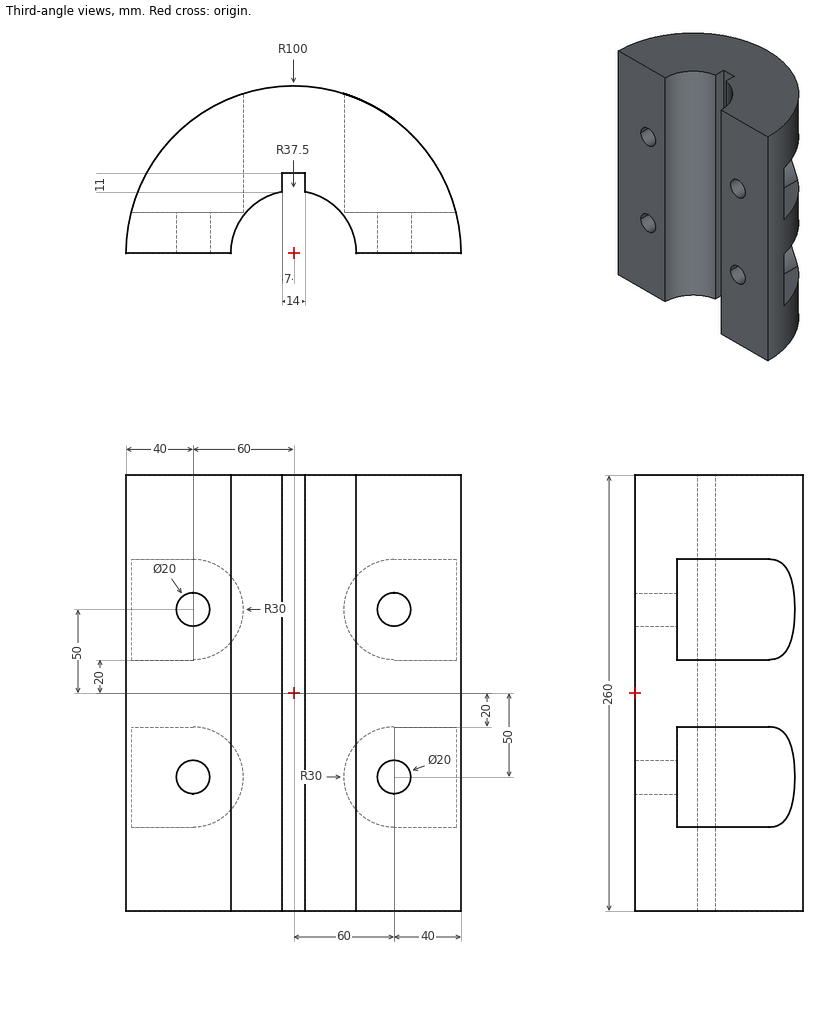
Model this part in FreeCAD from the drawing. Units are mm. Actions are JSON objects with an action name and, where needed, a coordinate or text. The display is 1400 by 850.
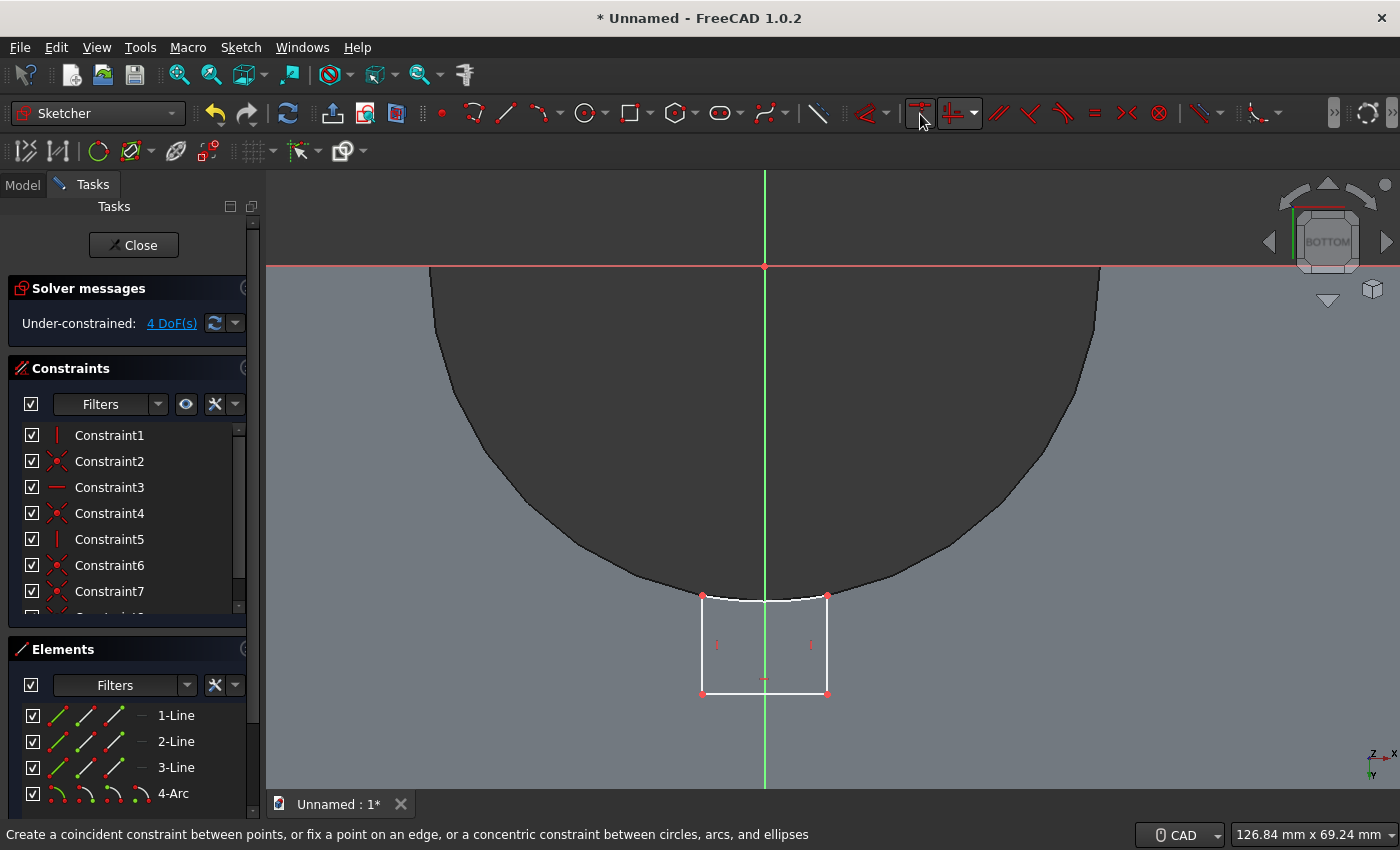
{"action": "left_click", "coordinate": [866, 114]}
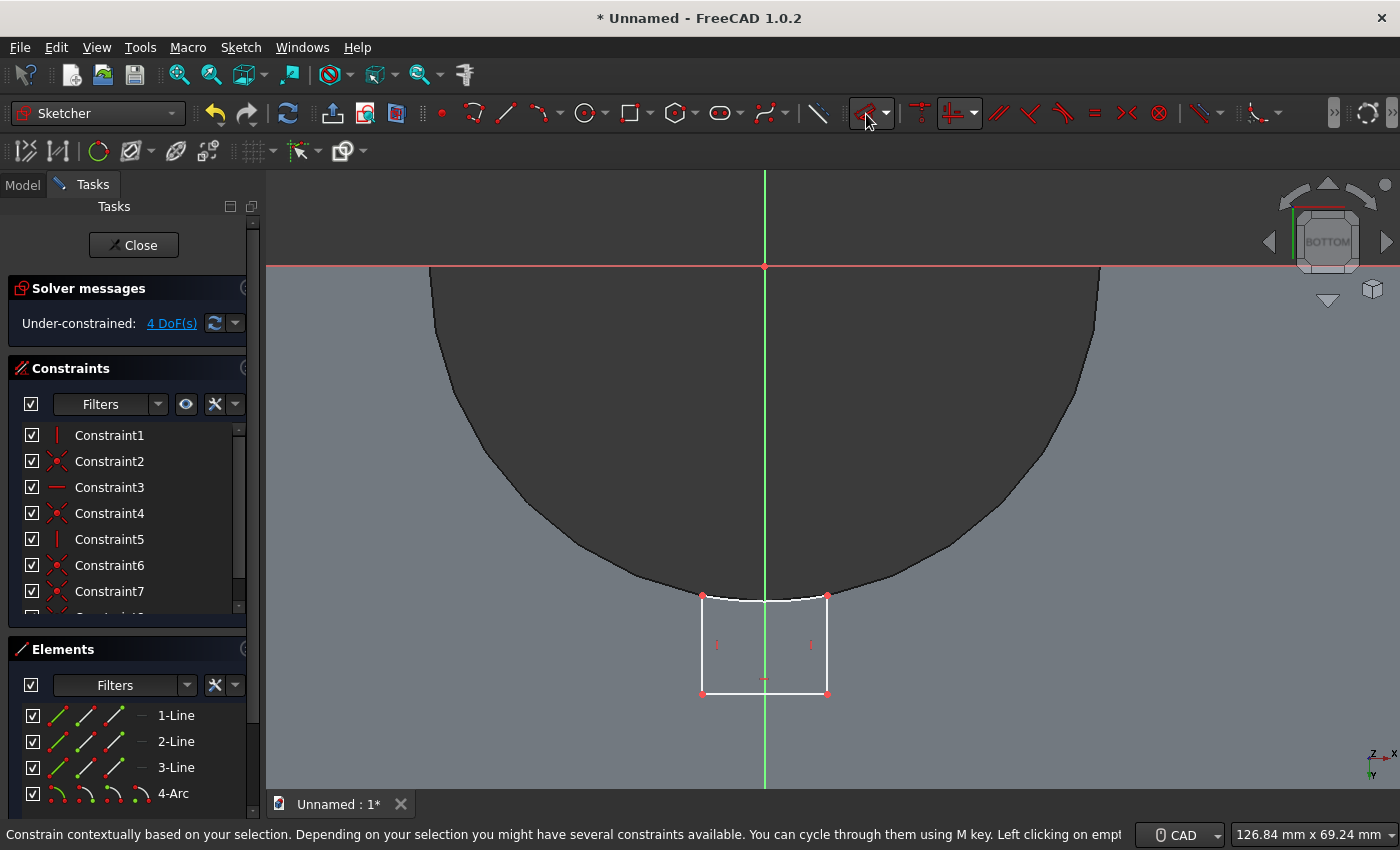
{"action": "left_click", "coordinate": [739, 601]}
{"action": "left_click", "coordinate": [737, 633]}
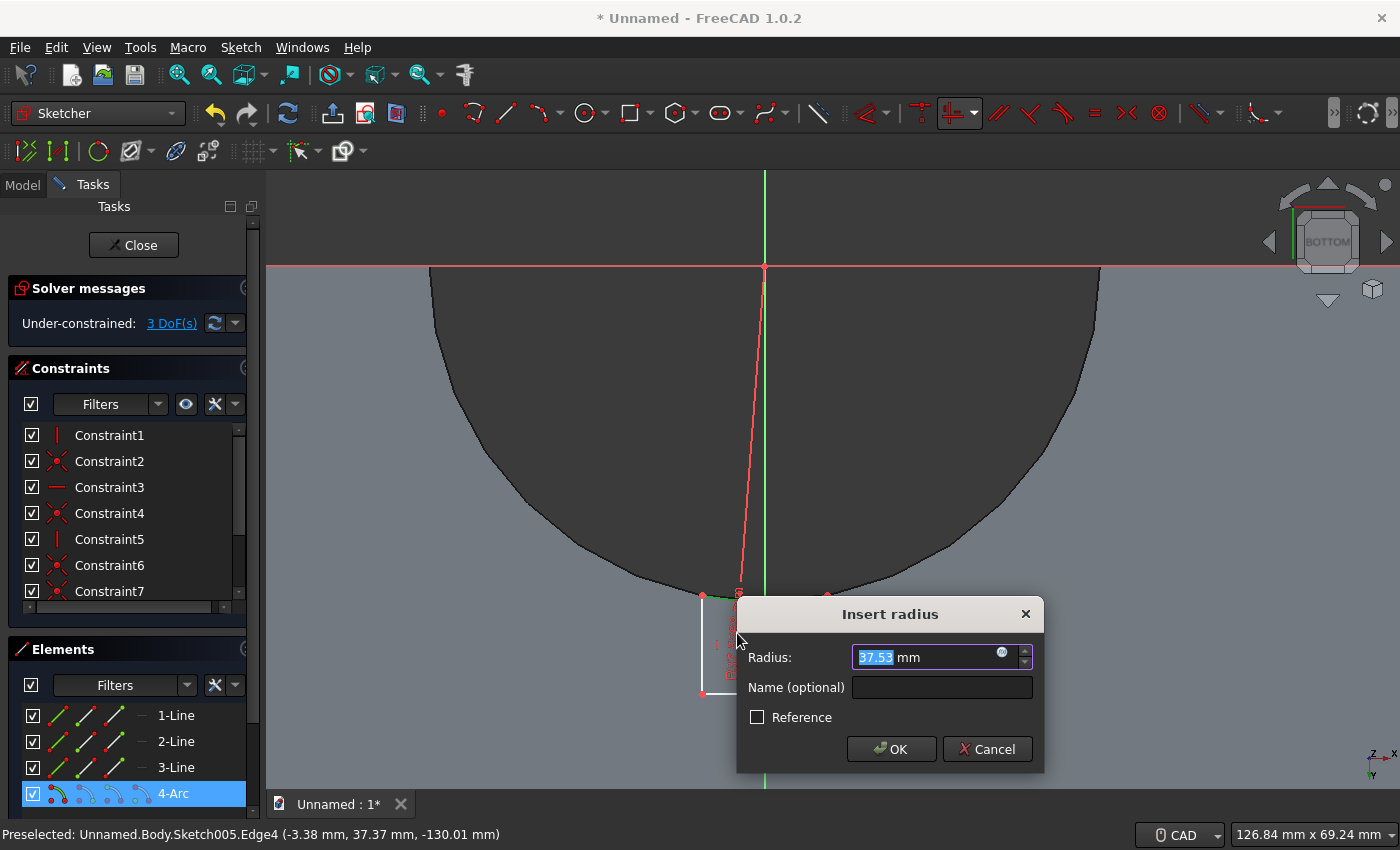
{"action": "type", "text": "37.5"}
{"action": "key", "text": "Return"}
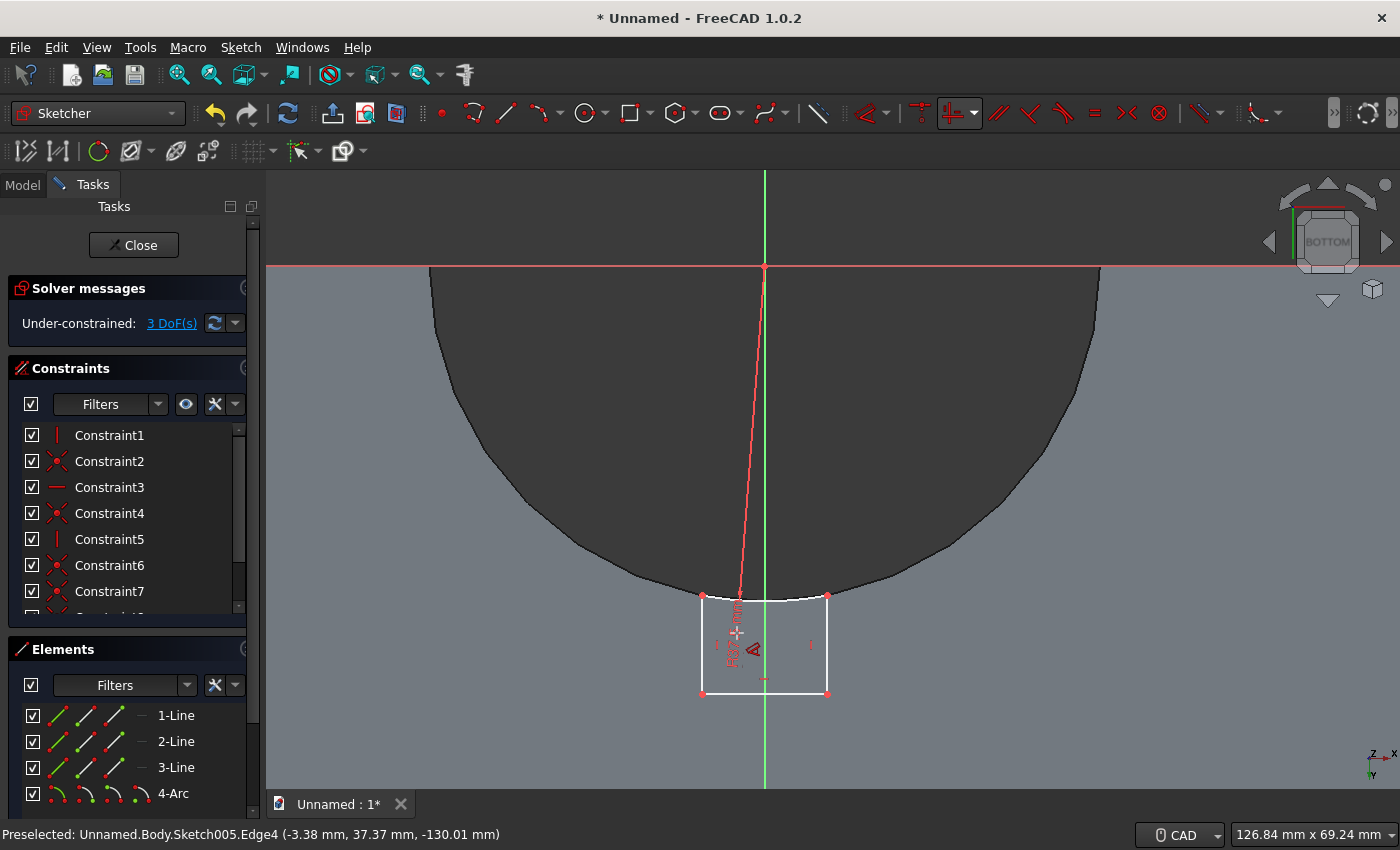
{"action": "left_click", "coordinate": [702, 625]}
{"action": "left_click", "coordinate": [668, 667]}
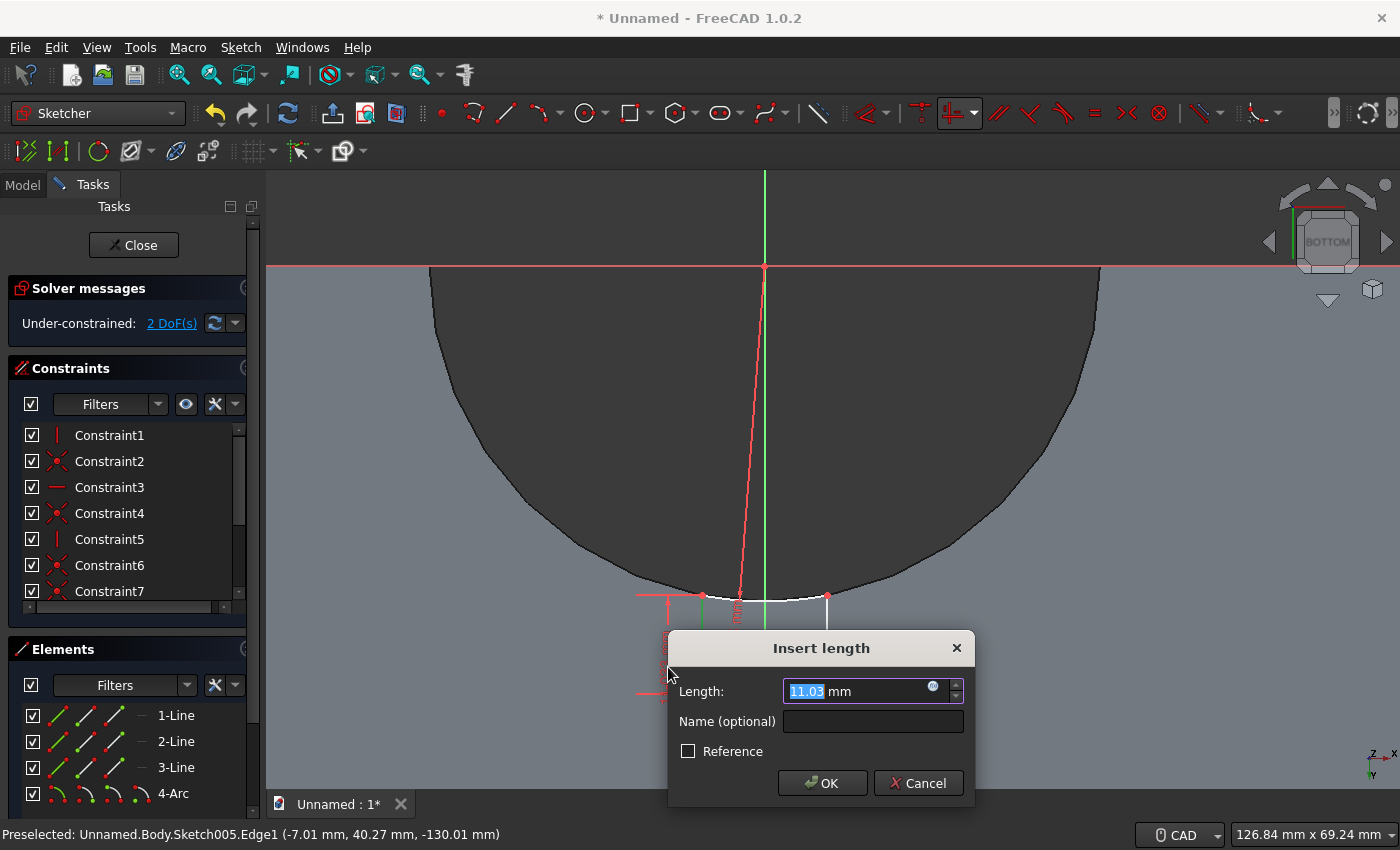
{"action": "type", "text": "11"}
{"action": "key", "text": "Return"}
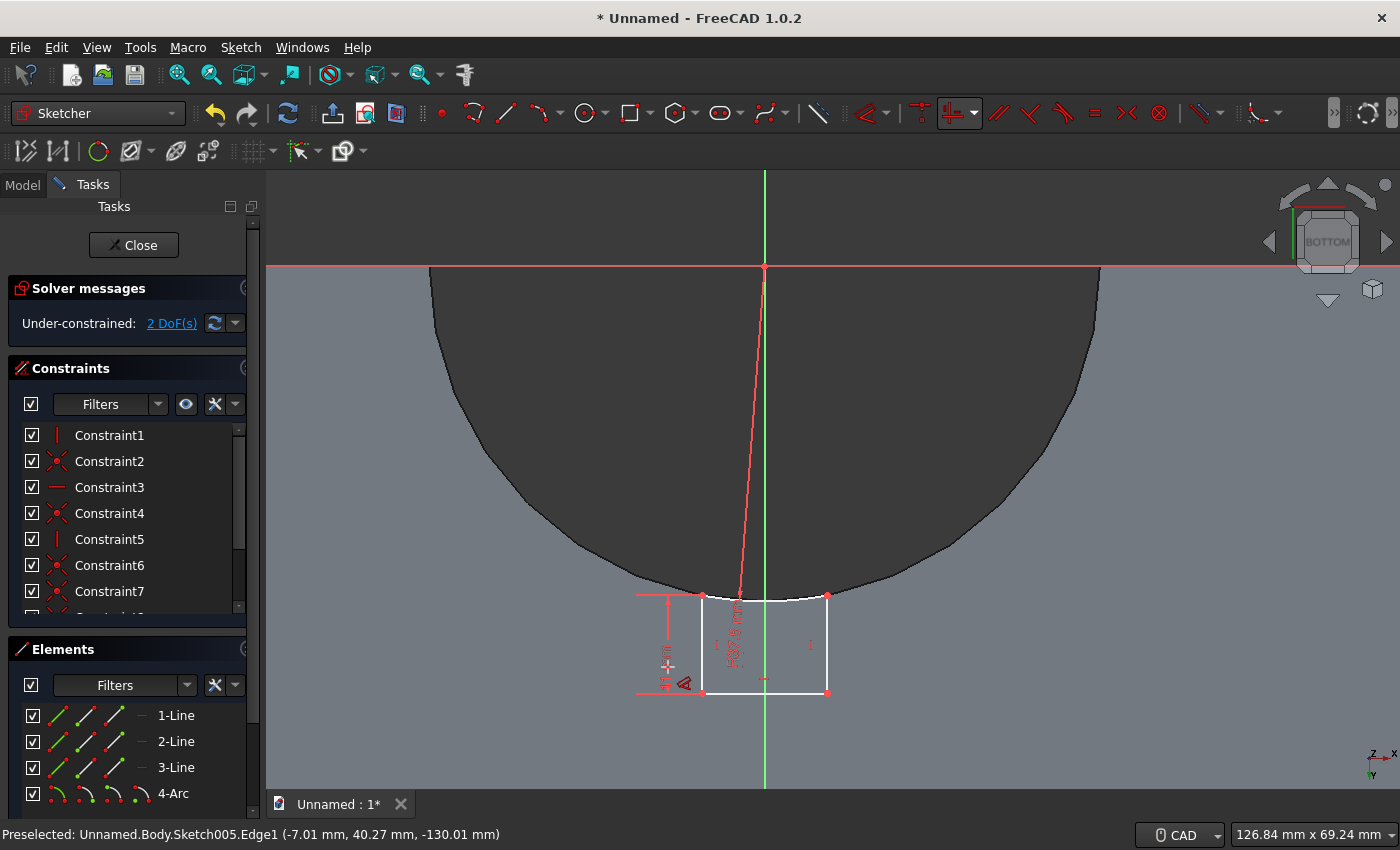
{"action": "left_click", "coordinate": [740, 694]}
{"action": "left_click", "coordinate": [736, 728]}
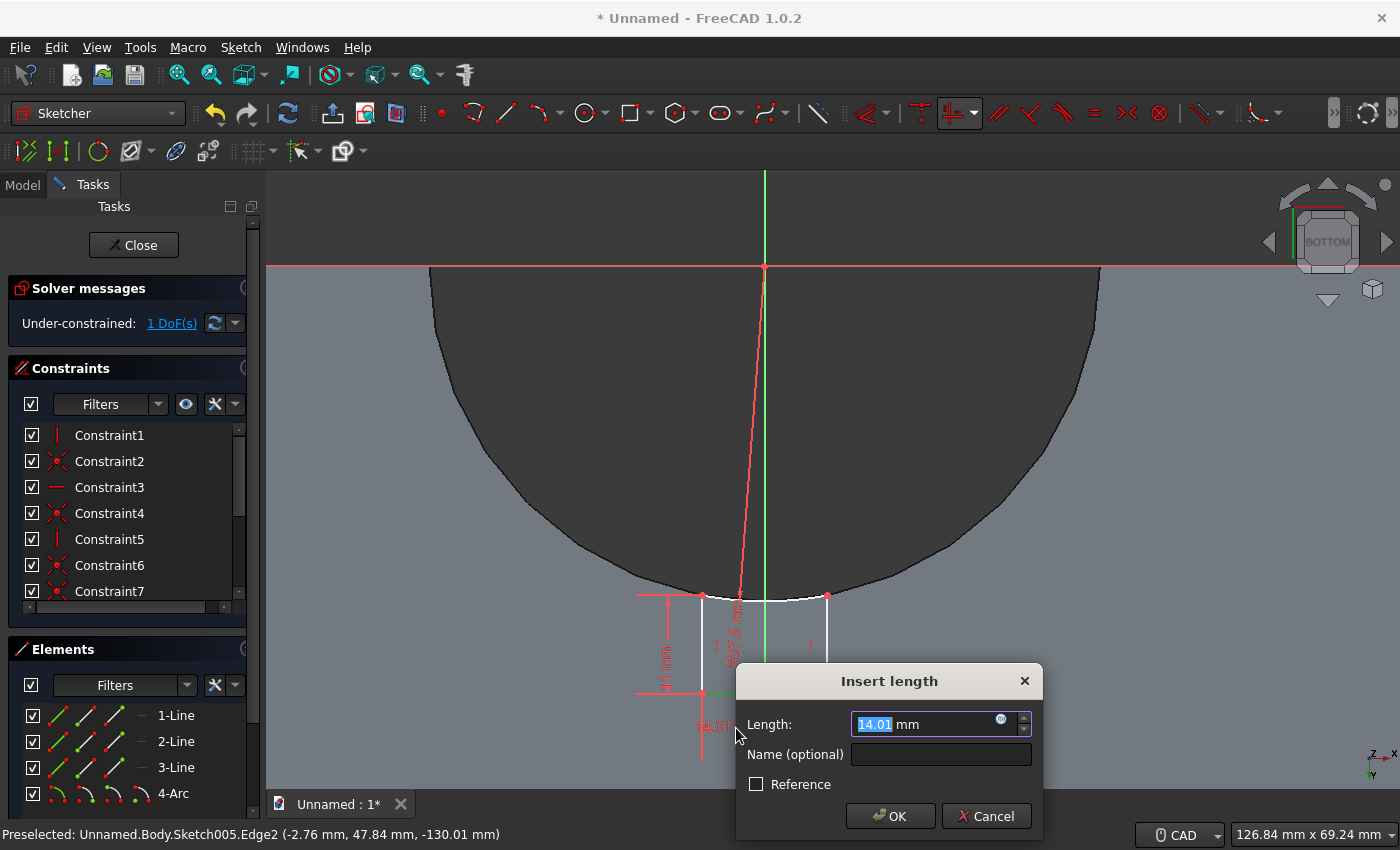
{"action": "type", "text": "14"}
{"action": "key", "text": "Return"}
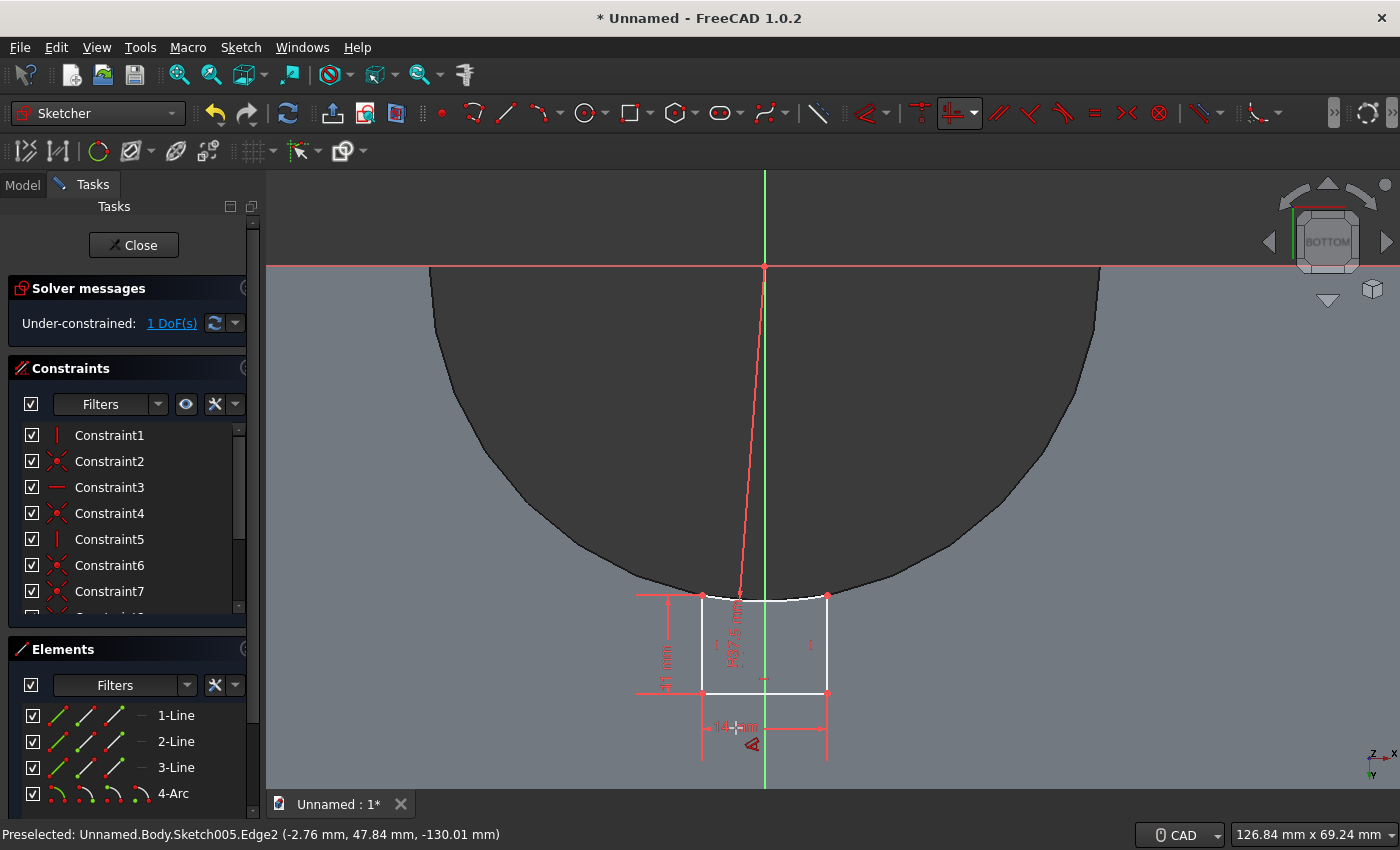
{"action": "left_click", "coordinate": [702, 595]}
{"action": "left_click", "coordinate": [733, 232]}